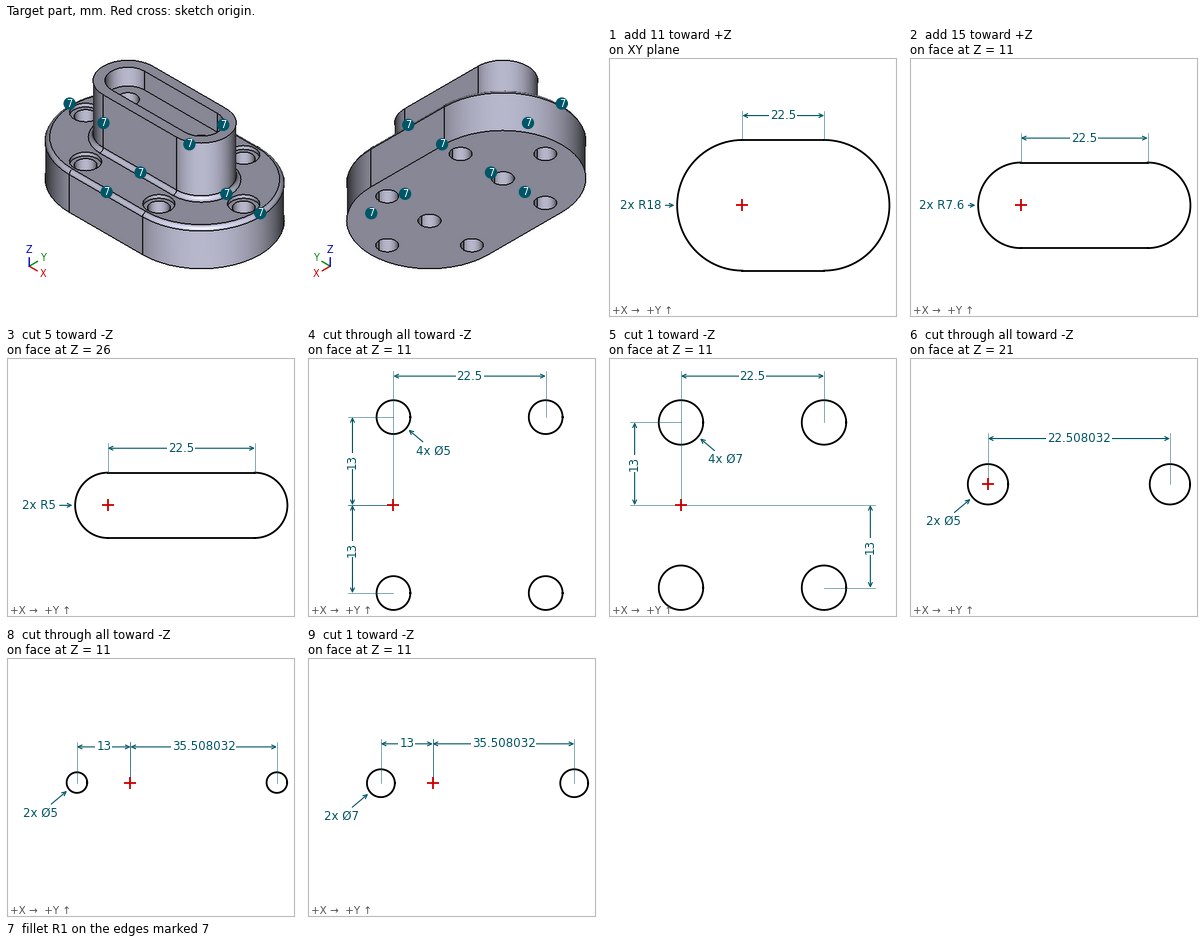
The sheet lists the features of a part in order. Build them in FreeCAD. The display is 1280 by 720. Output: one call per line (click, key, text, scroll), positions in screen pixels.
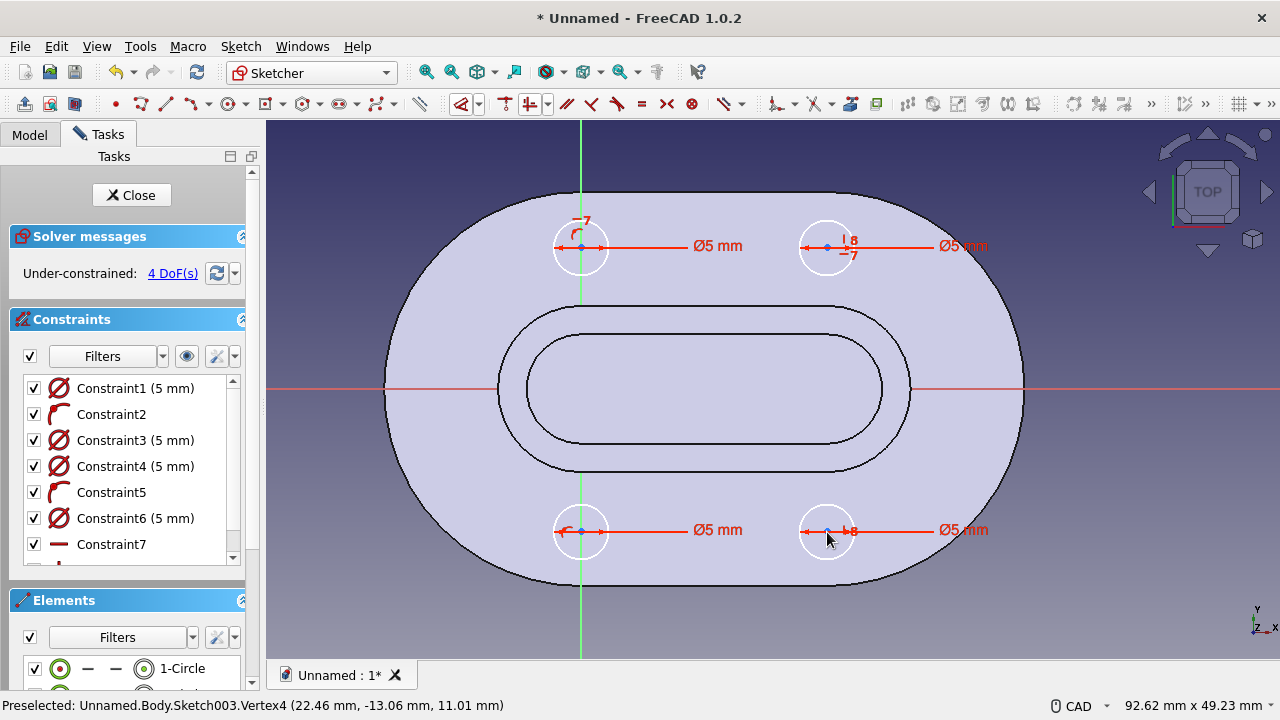
click(581, 532)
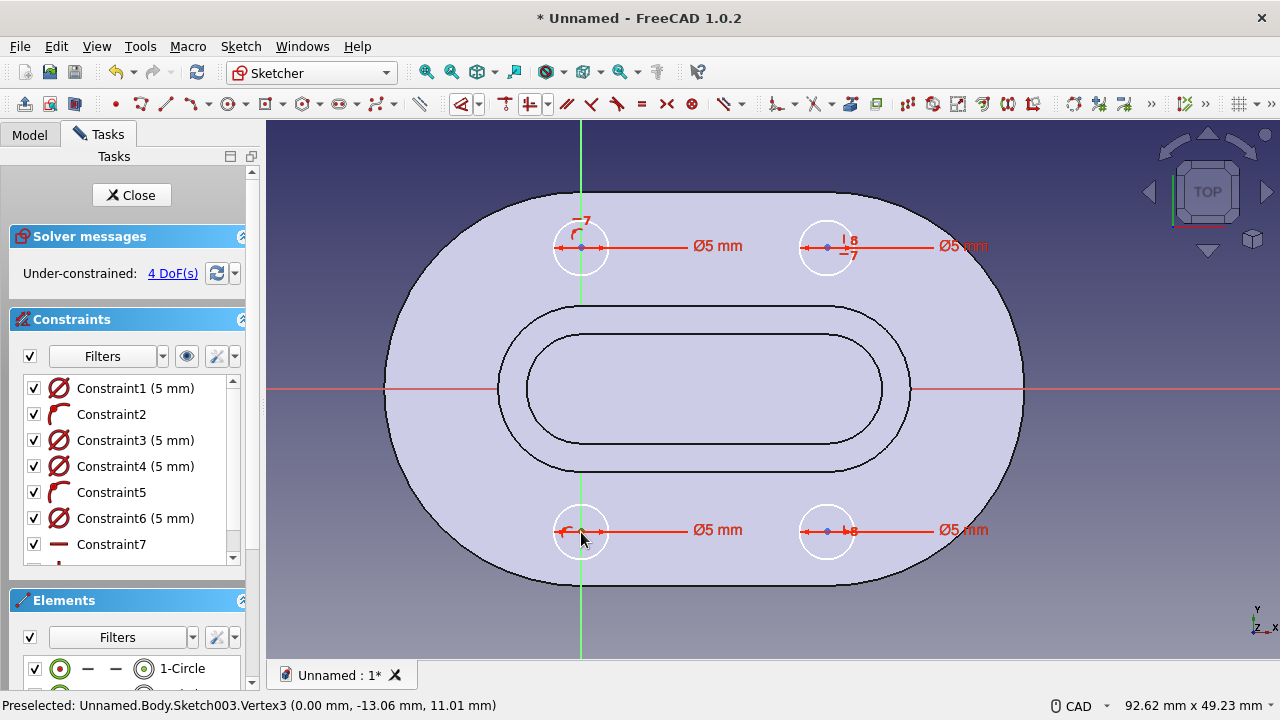
click(827, 532)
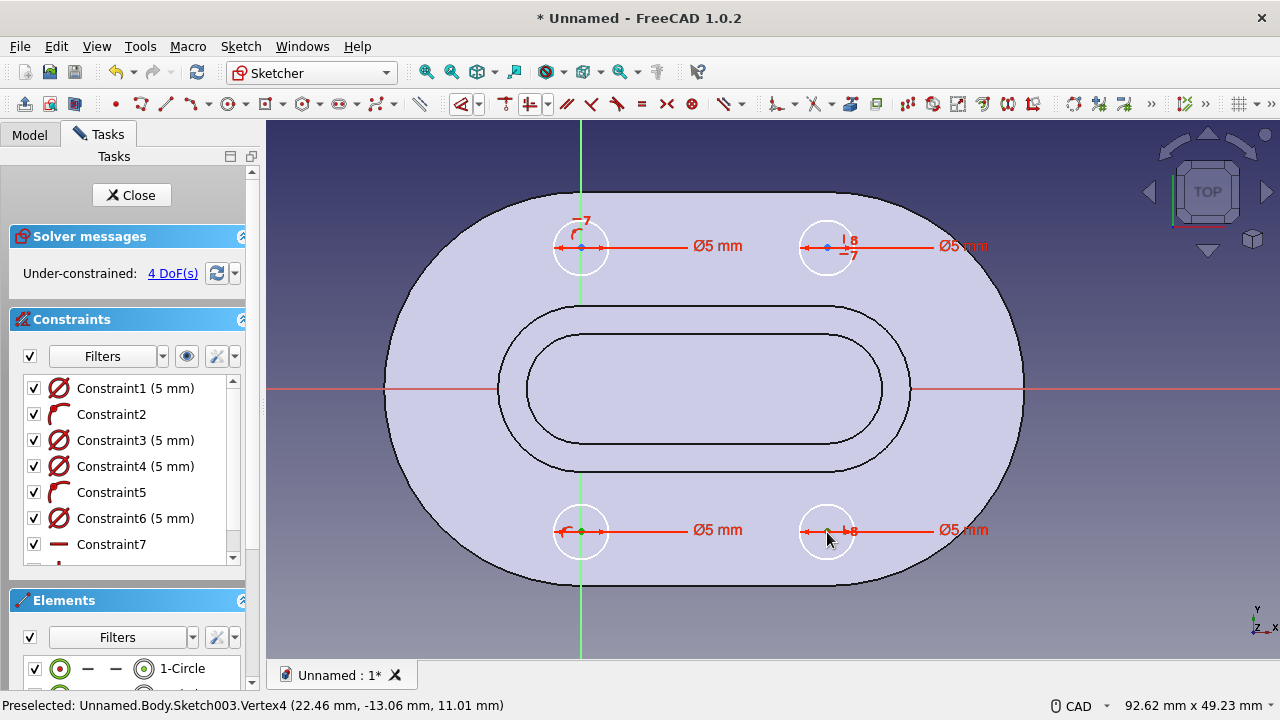
click(548, 104)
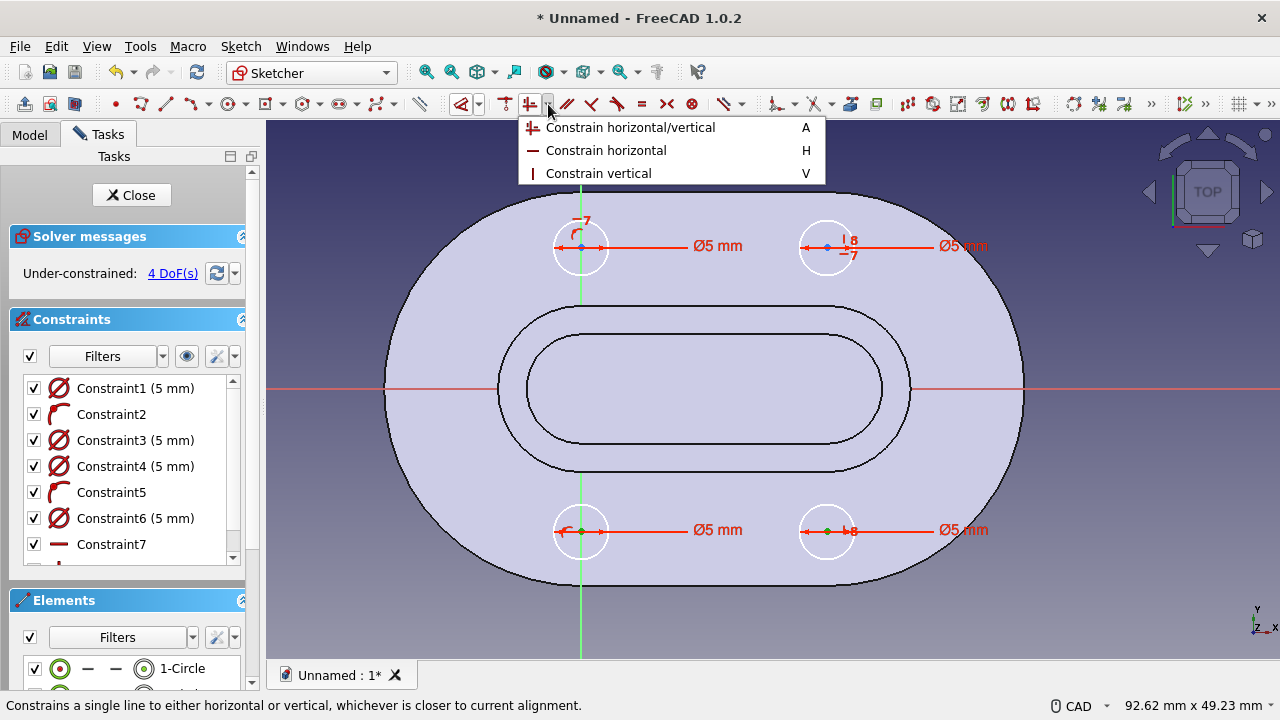
click(672, 150)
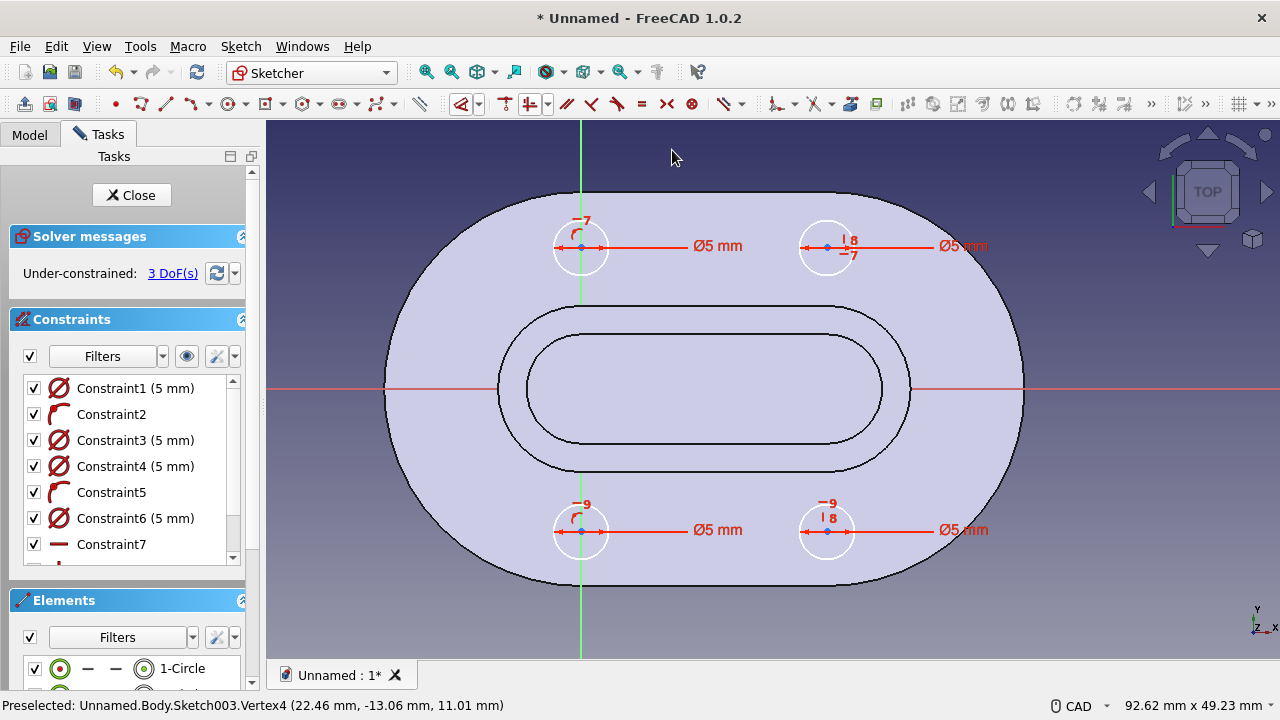
click(581, 248)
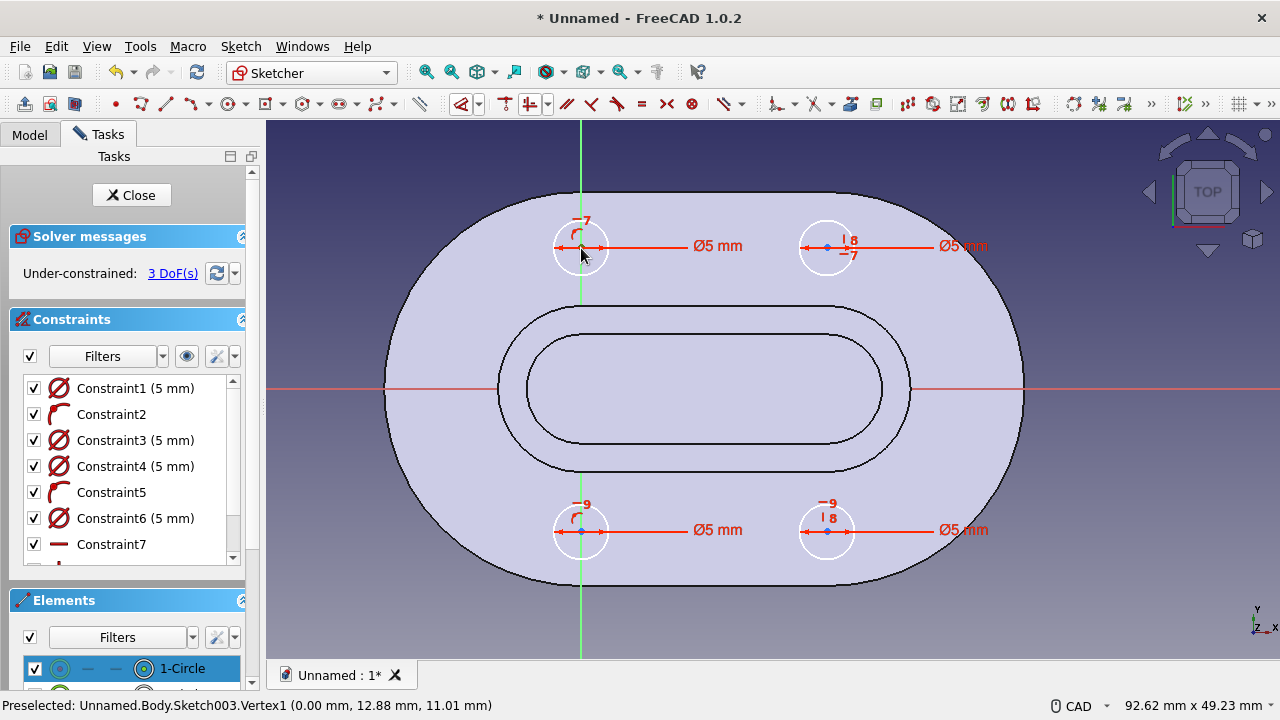
key(i)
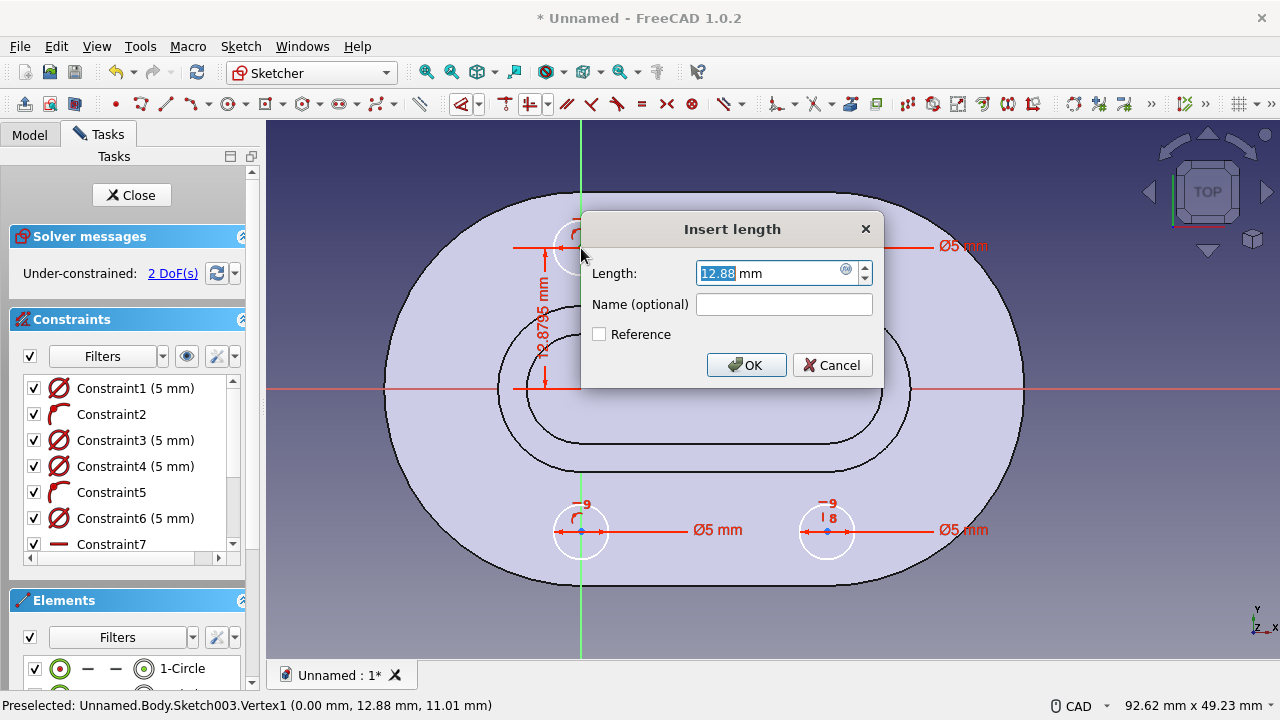
text(13)
key(Return)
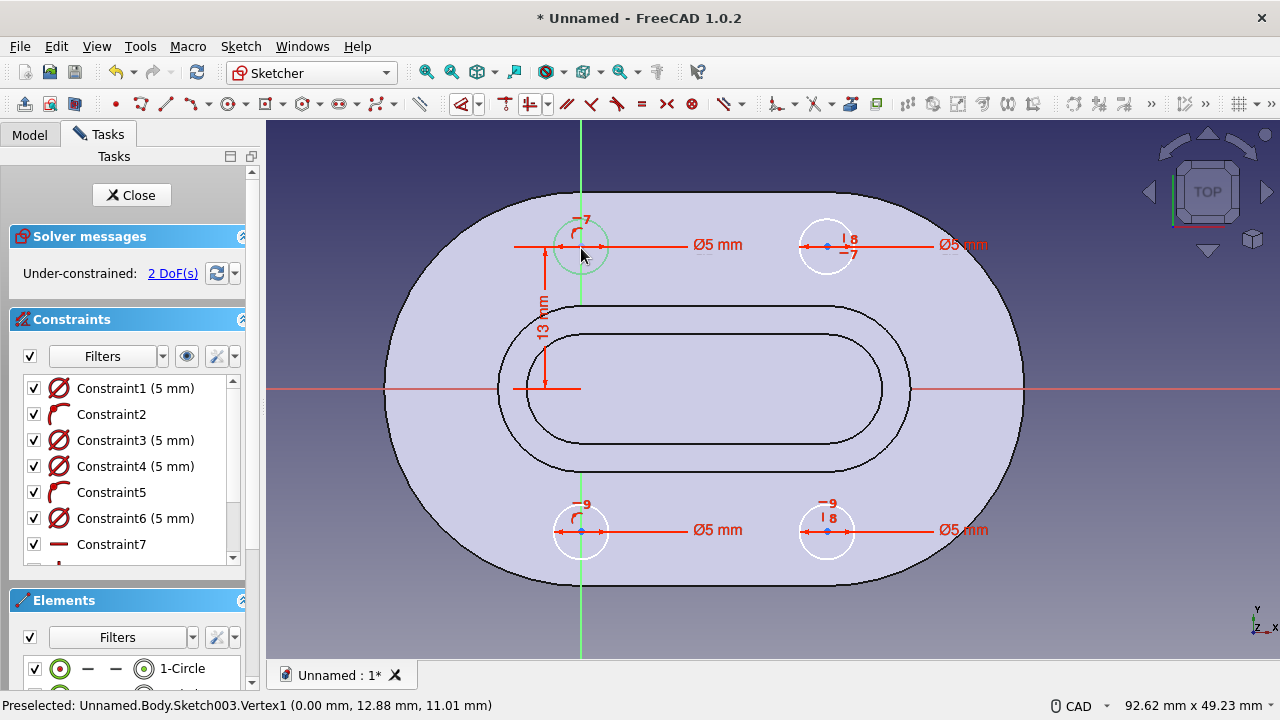
click(581, 532)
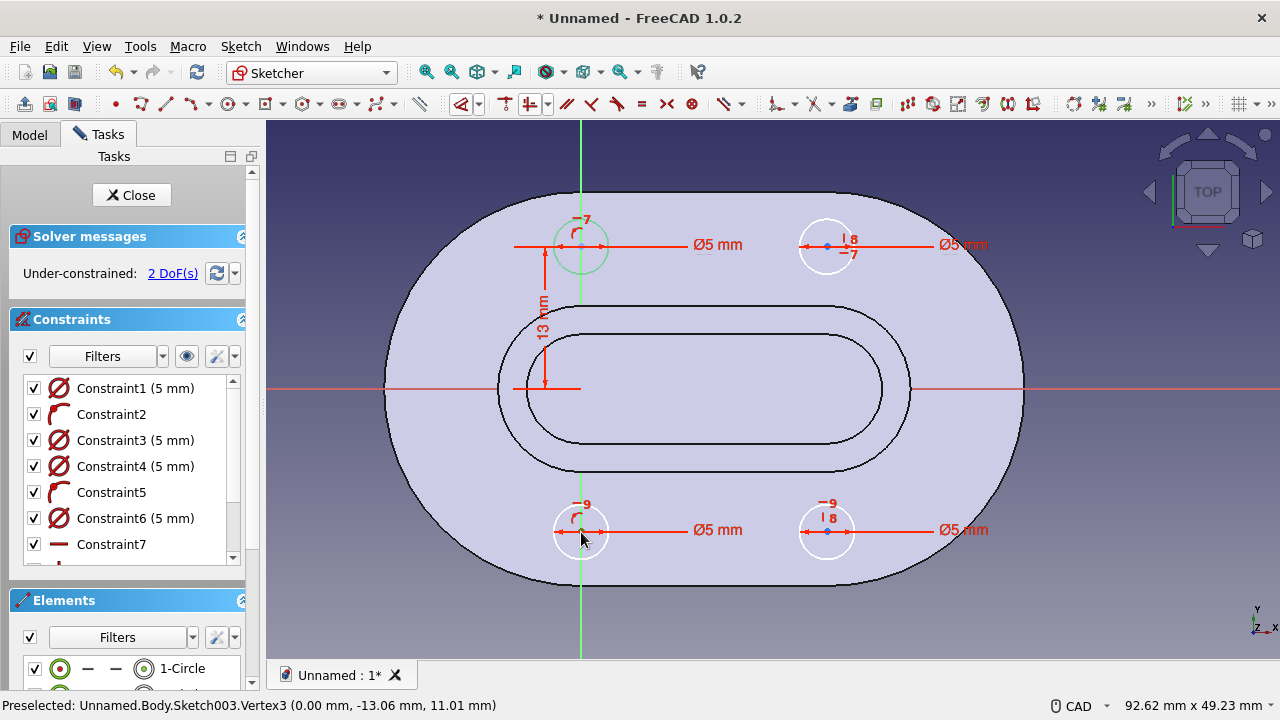
key(i)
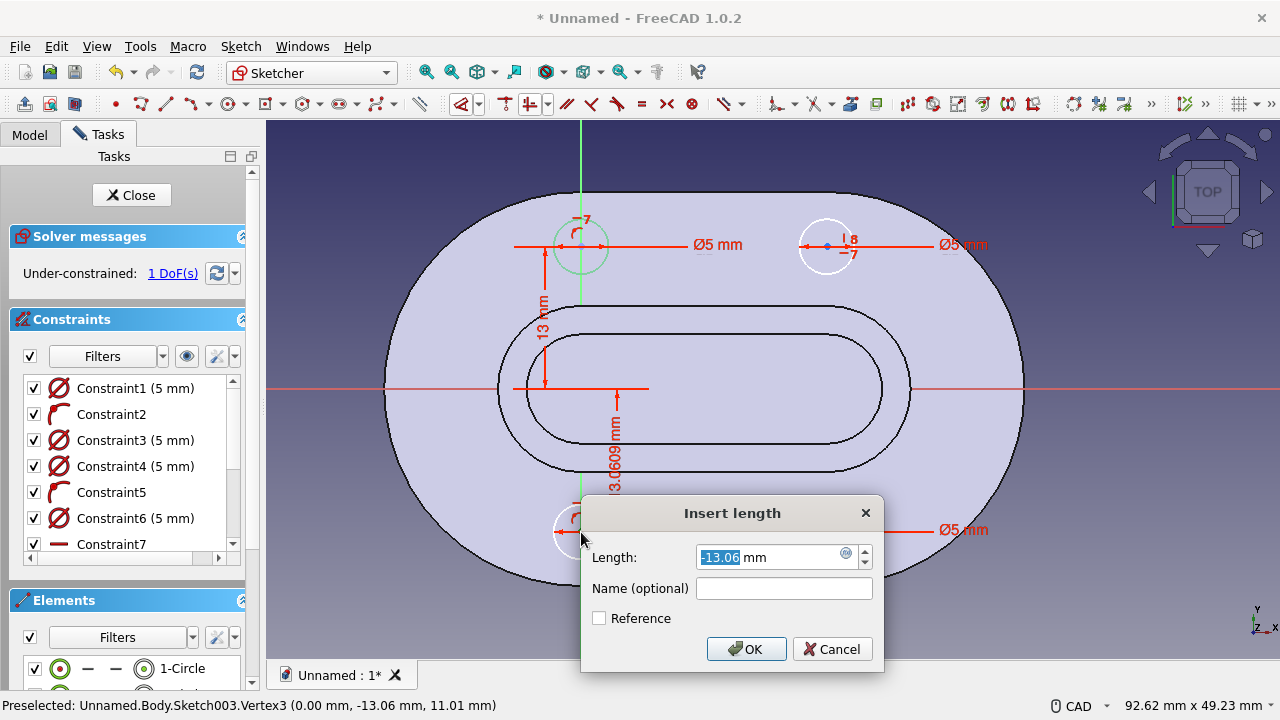
text(-13)
key(Return)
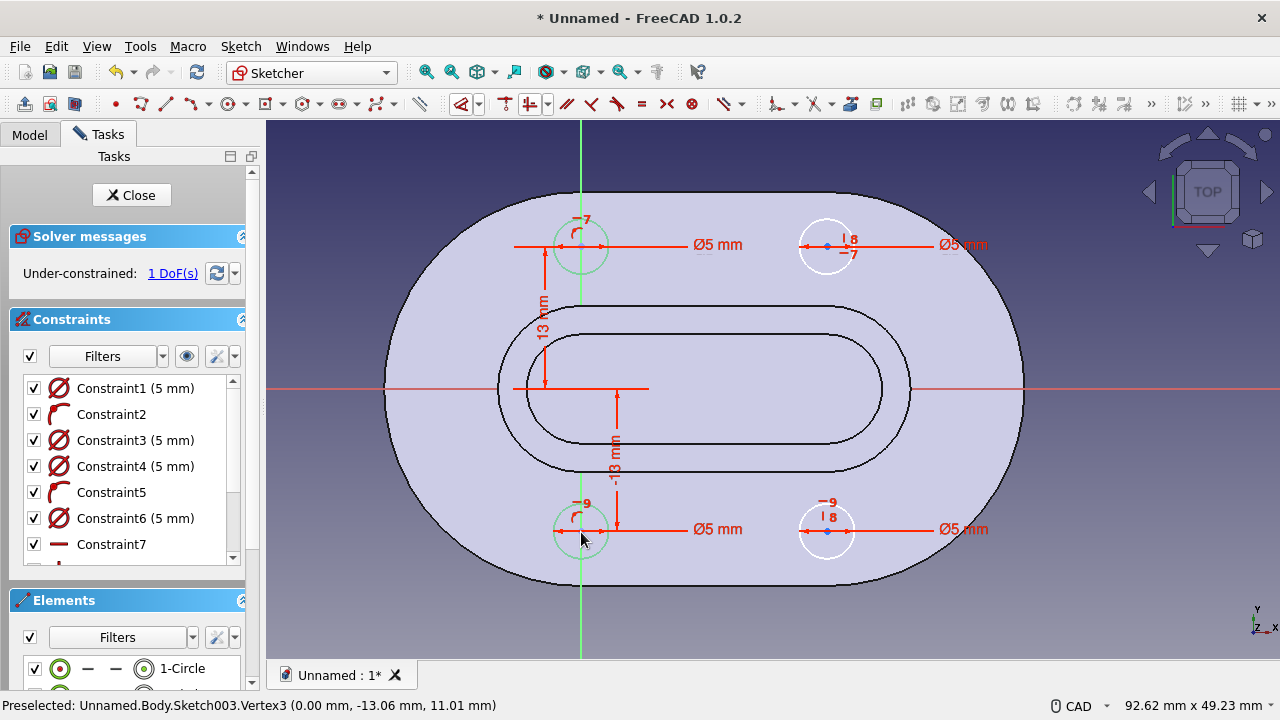
click(827, 247)